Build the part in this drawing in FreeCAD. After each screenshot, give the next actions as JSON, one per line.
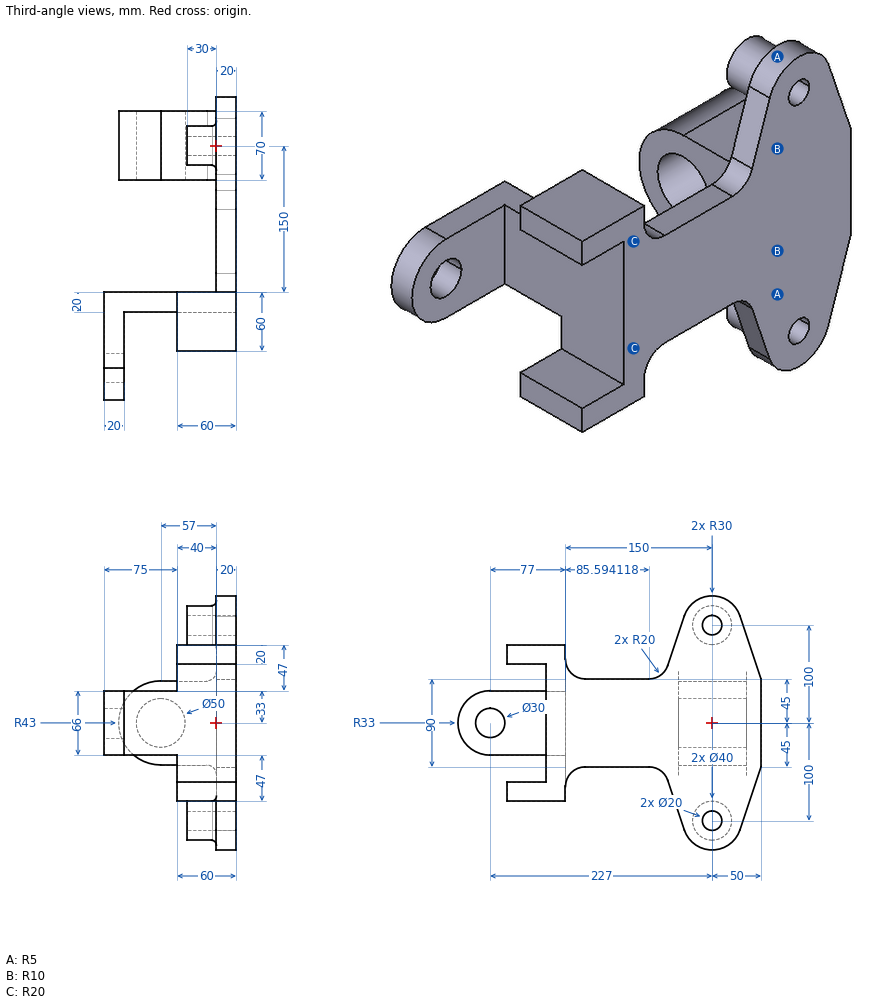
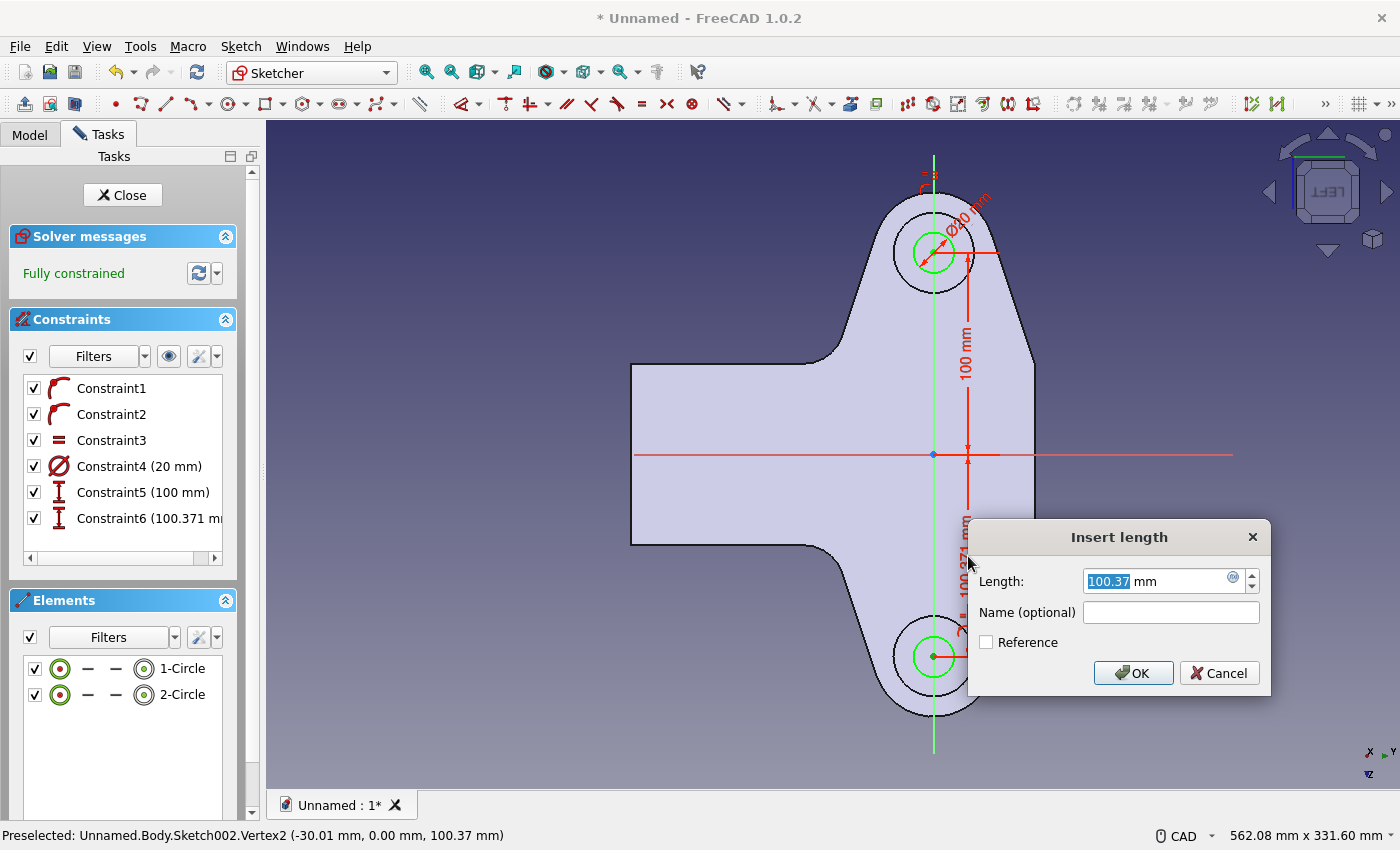
{"action": "type", "text": "100"}
{"action": "key", "text": "Return"}
{"action": "key", "text": "Escape"}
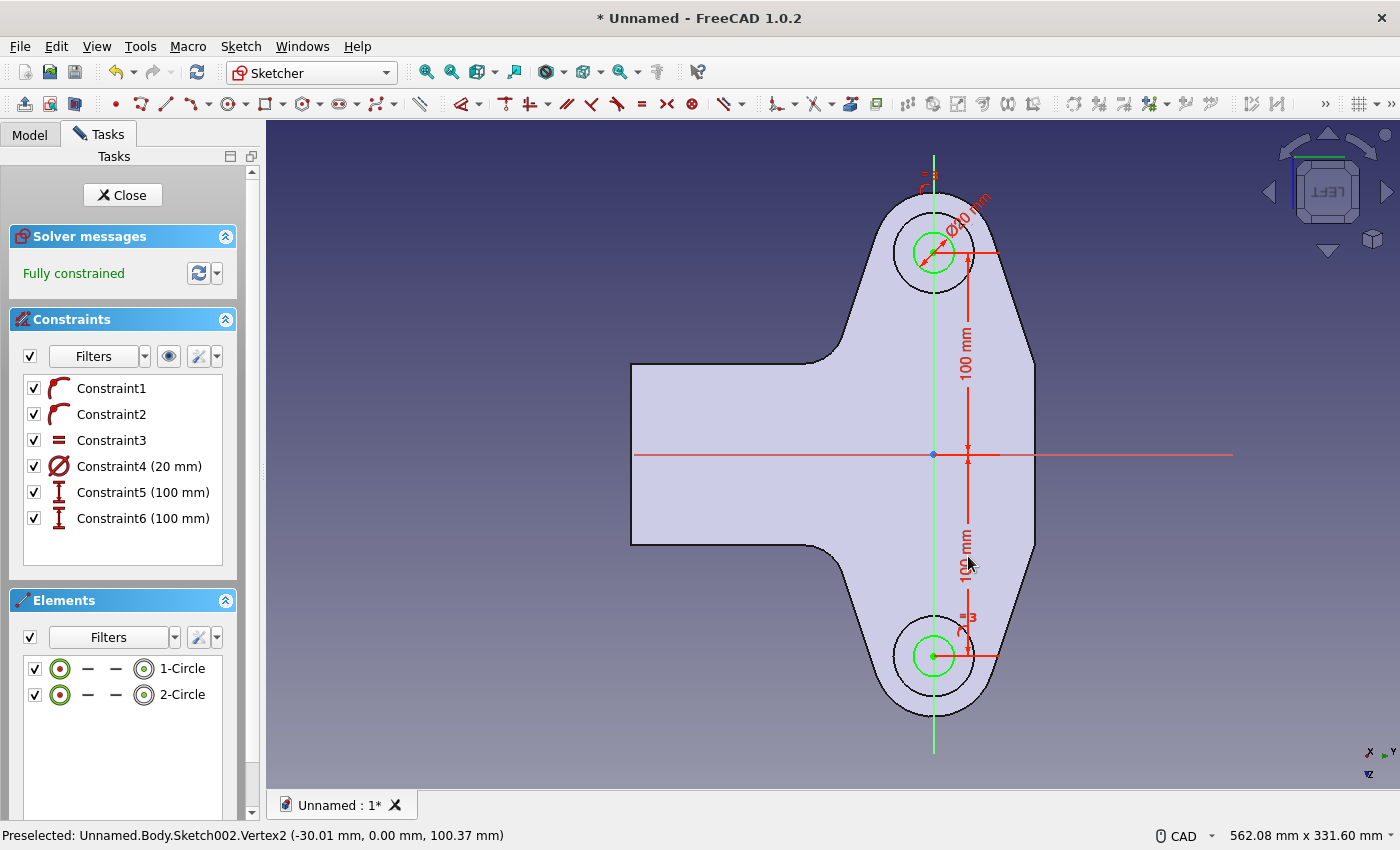
{"action": "left_click", "coordinate": [123, 195]}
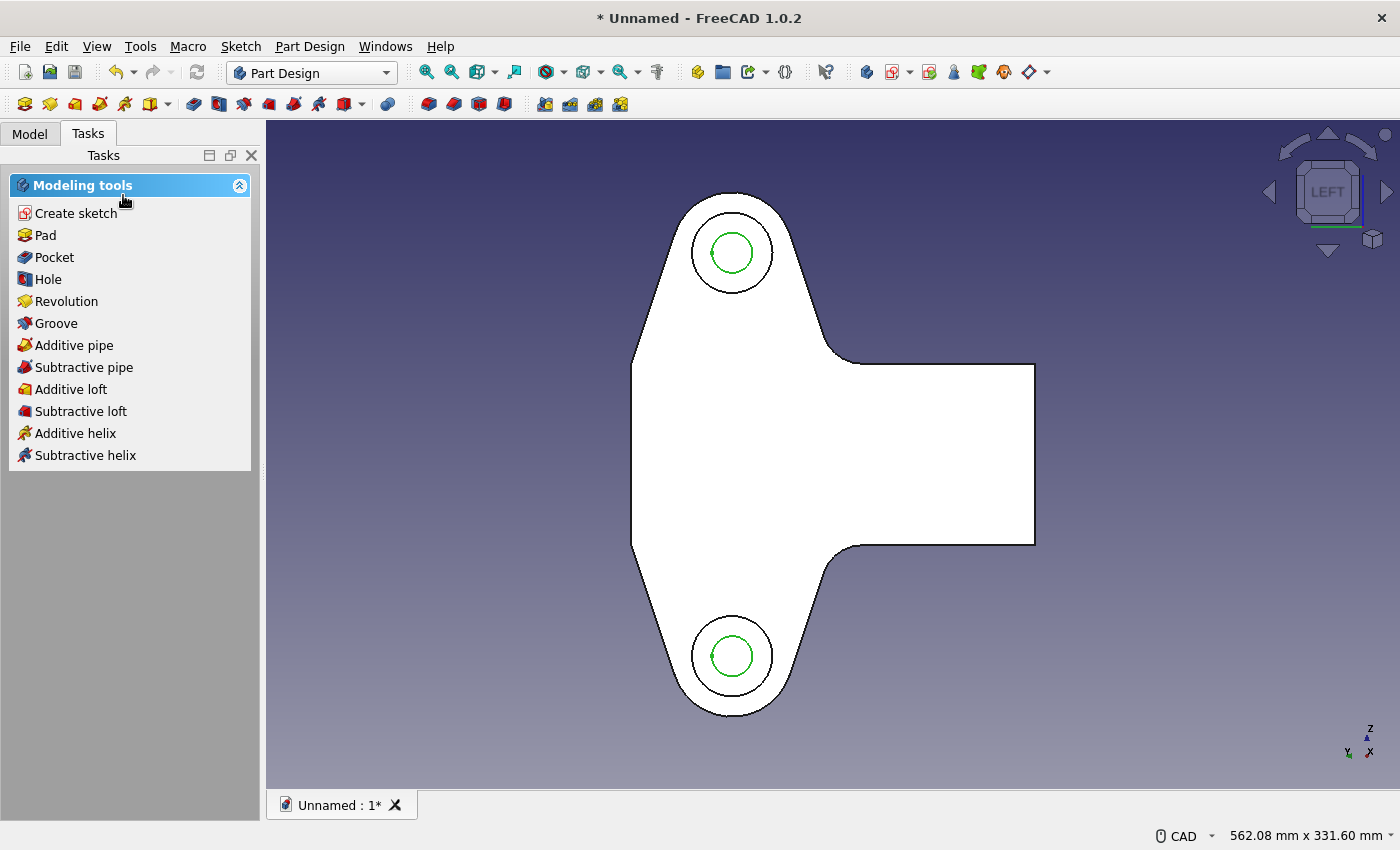
{"action": "left_click", "coordinate": [194, 104]}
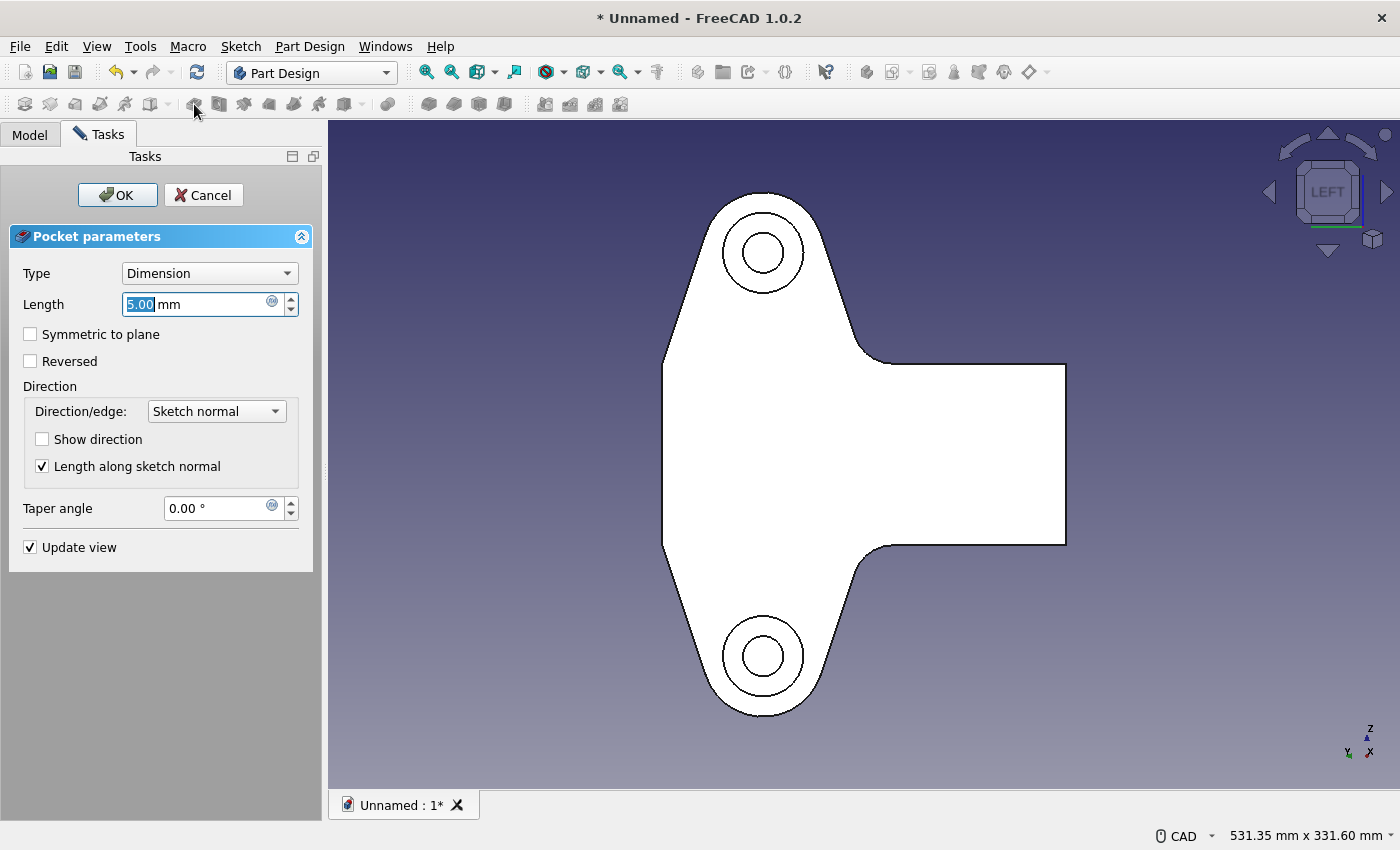
{"action": "left_click", "coordinate": [210, 274]}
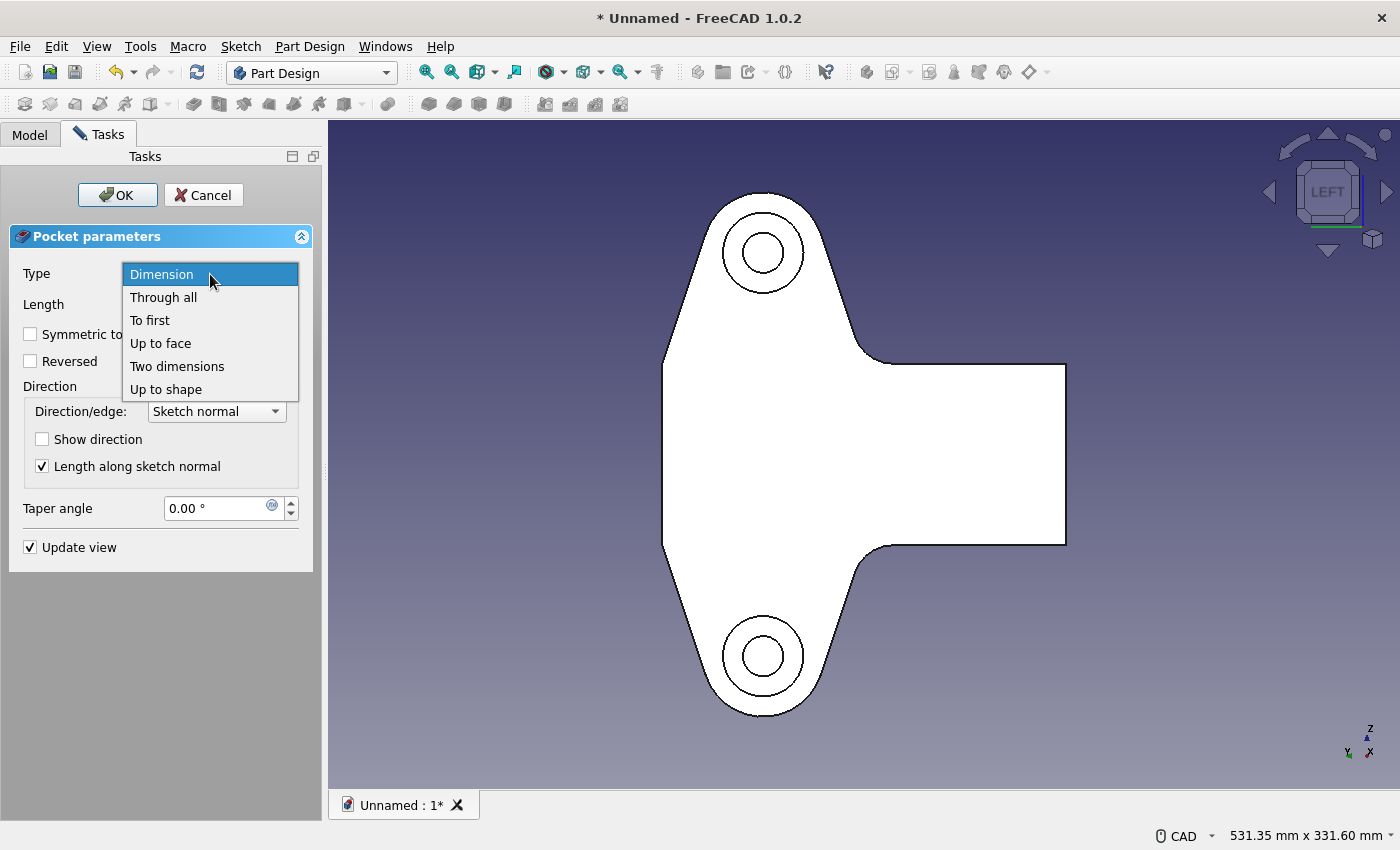
{"action": "left_click", "coordinate": [208, 298]}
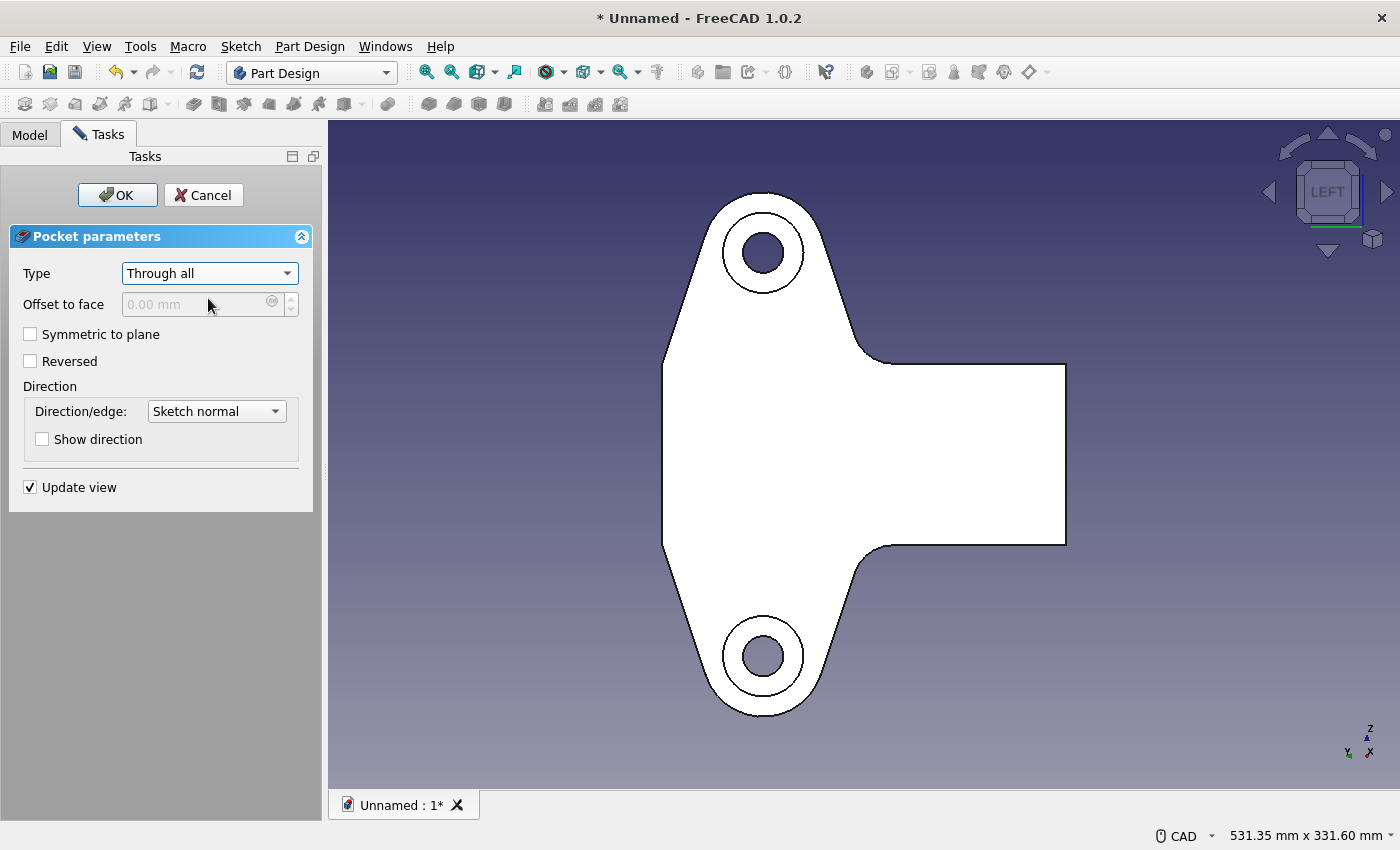
{"action": "left_click", "coordinate": [118, 195]}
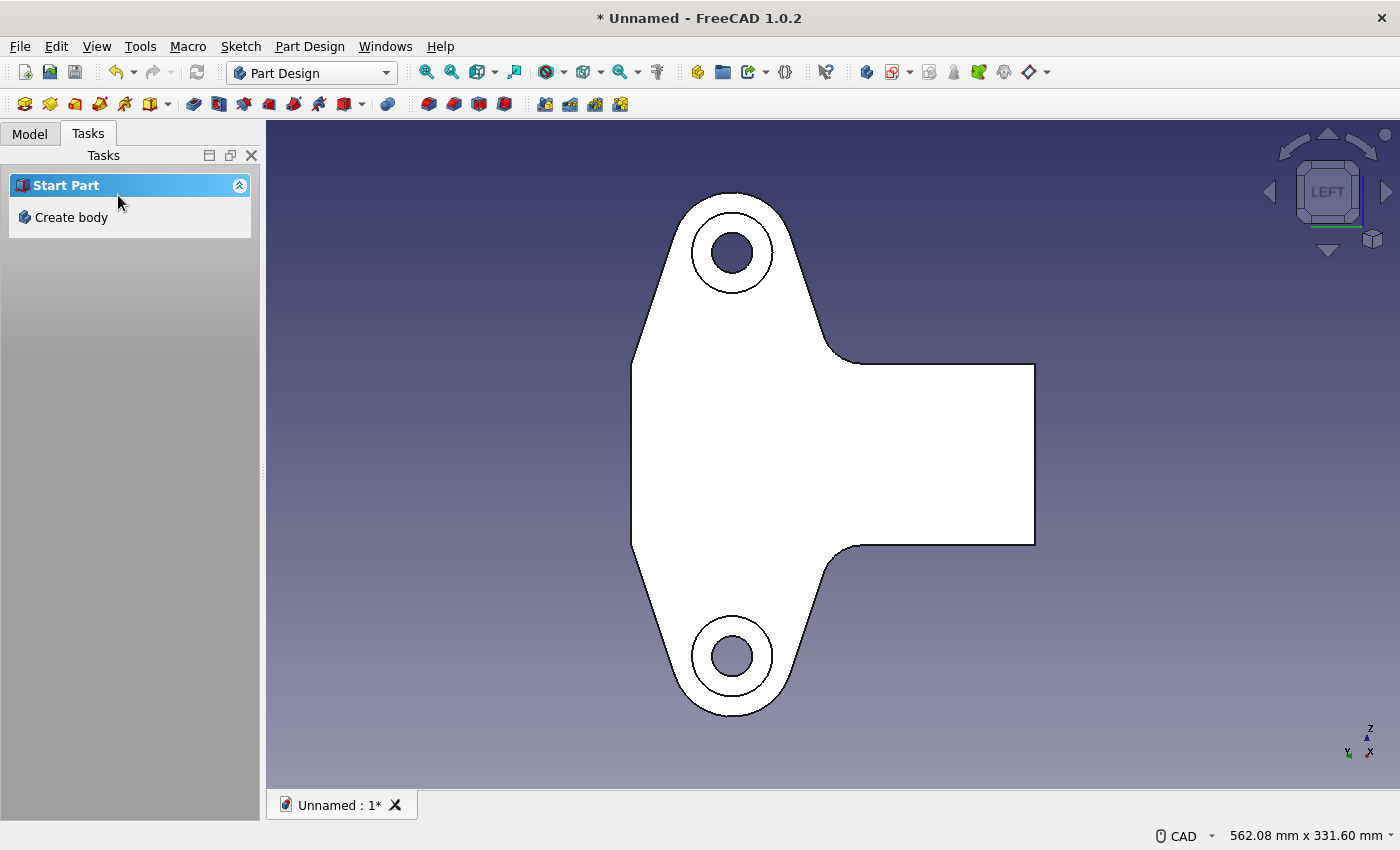
{"action": "left_click", "coordinate": [892, 72]}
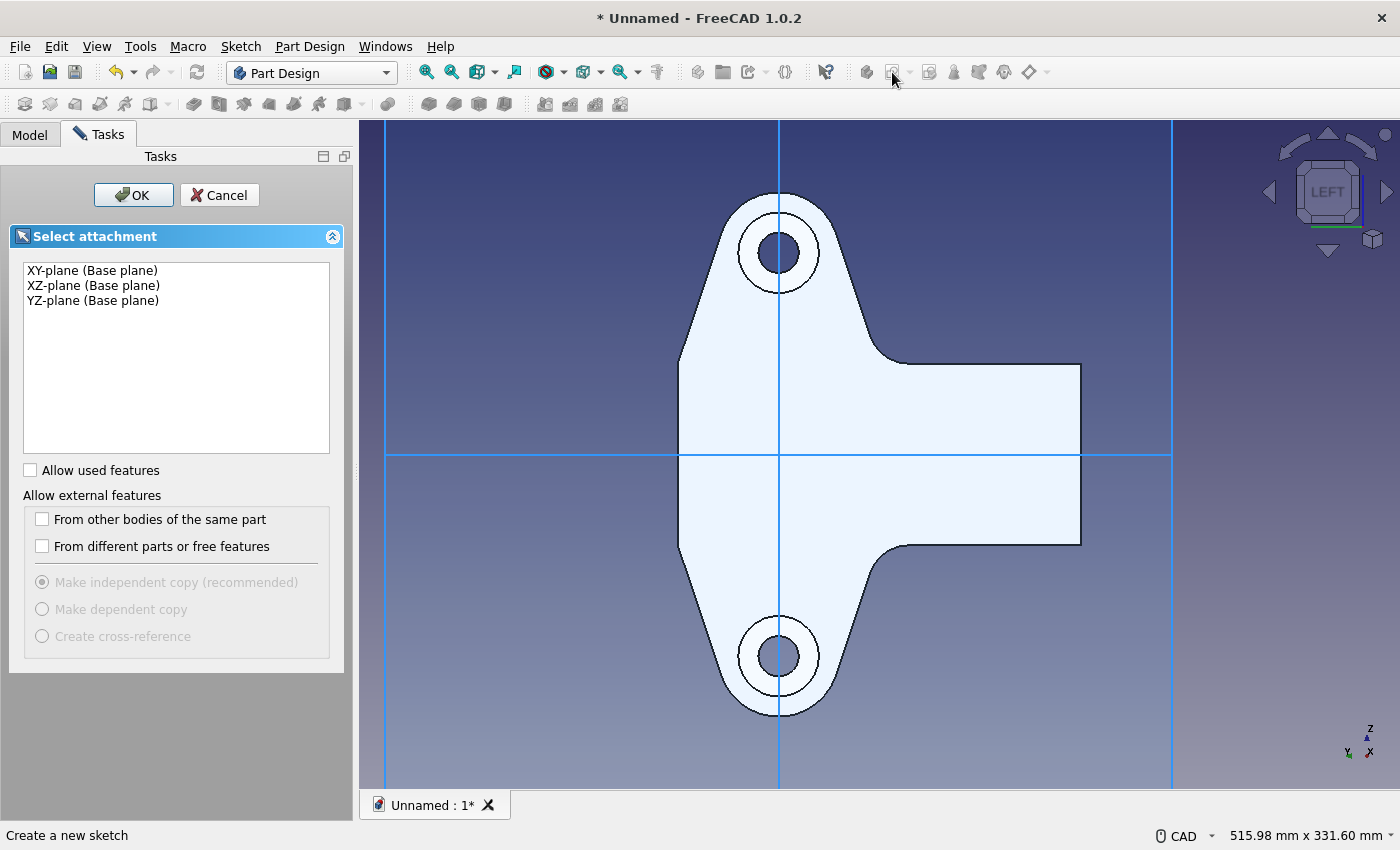
{"action": "left_click", "coordinate": [84, 286]}